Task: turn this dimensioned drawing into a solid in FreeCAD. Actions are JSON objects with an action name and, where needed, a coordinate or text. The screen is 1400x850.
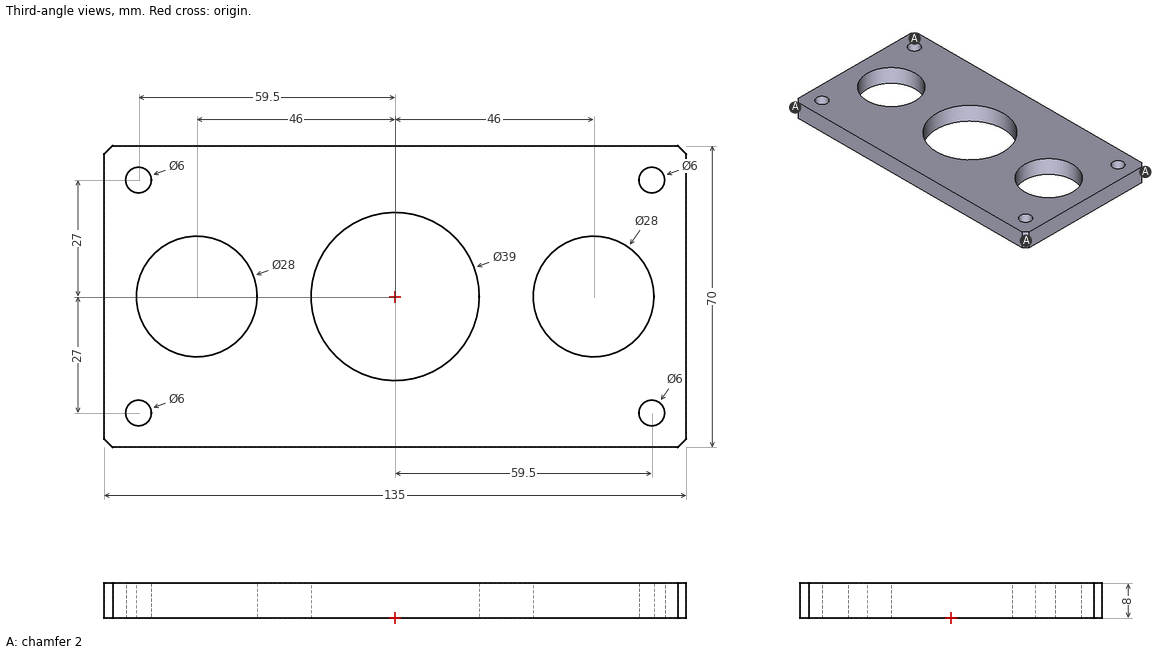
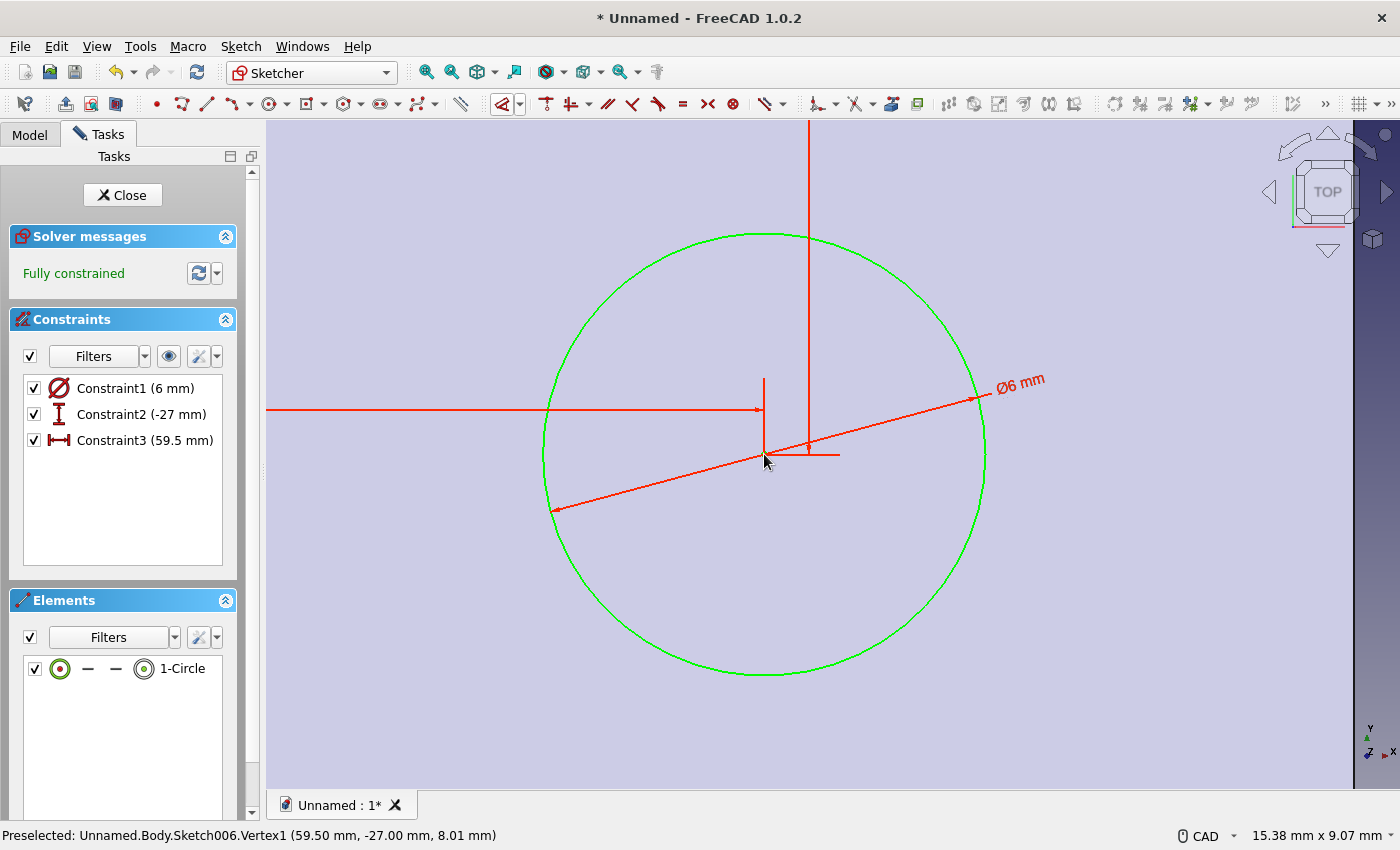
{"action": "left_click", "coordinate": [123, 195]}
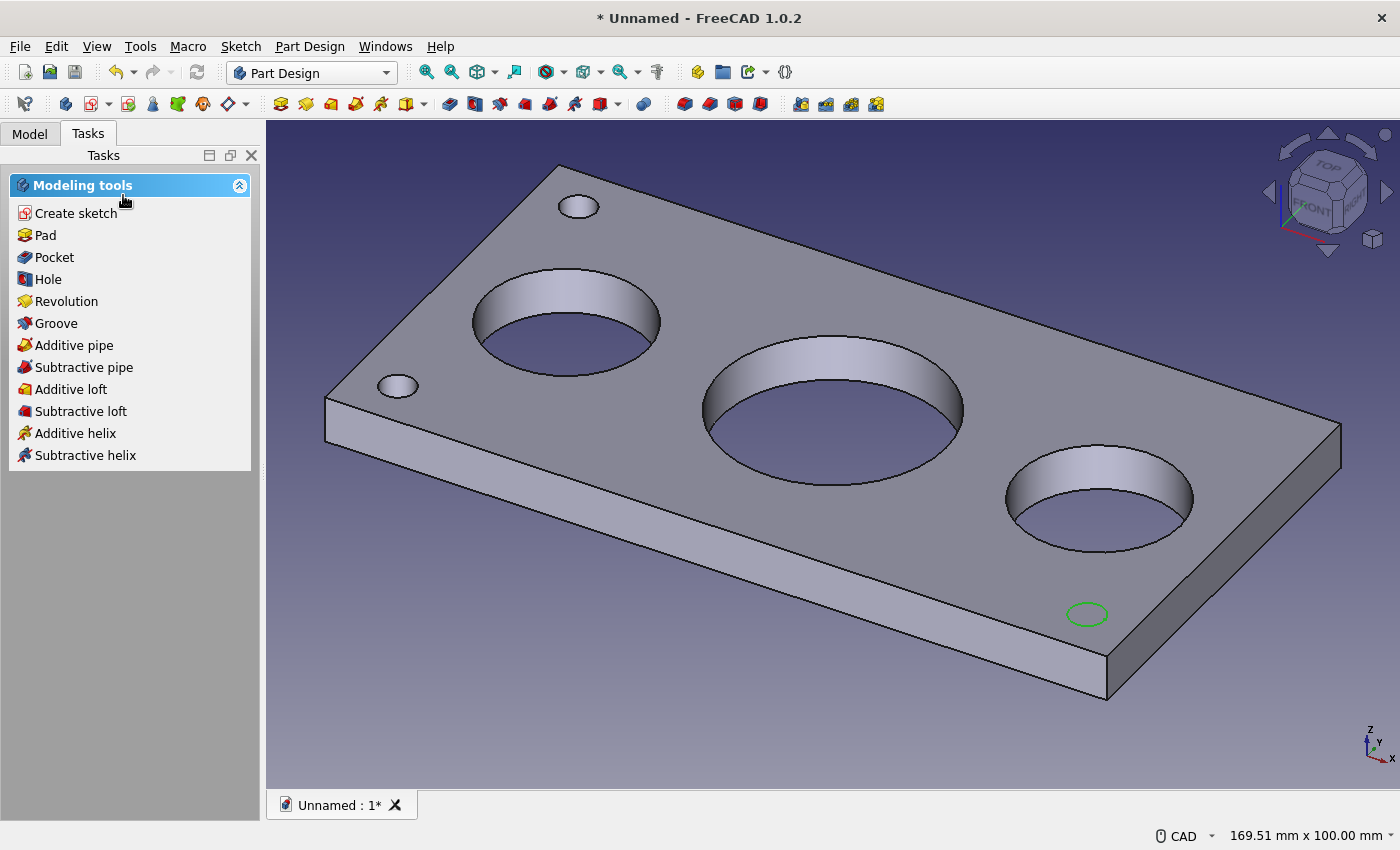
{"action": "left_click", "coordinate": [450, 104]}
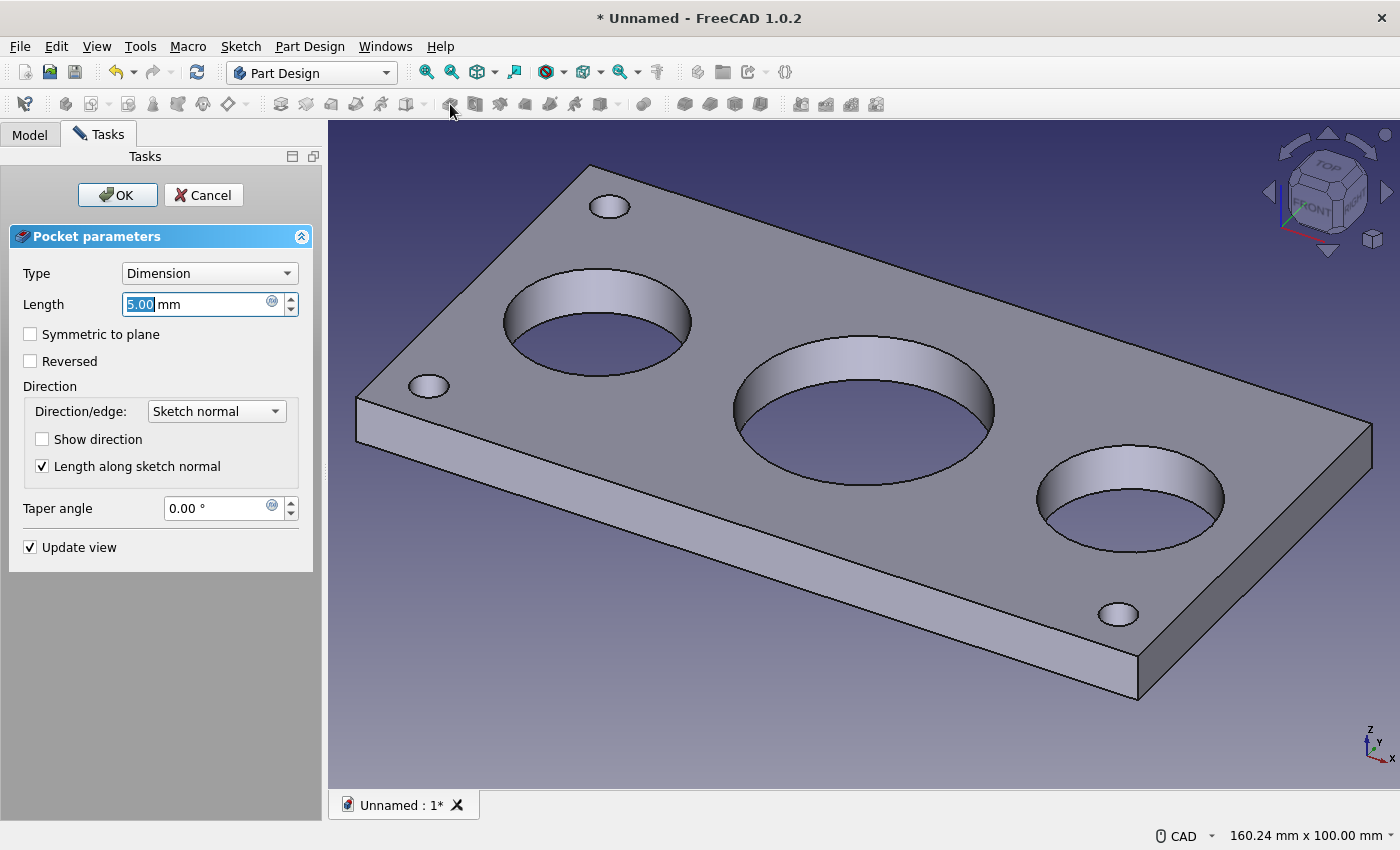
{"action": "left_click", "coordinate": [210, 274]}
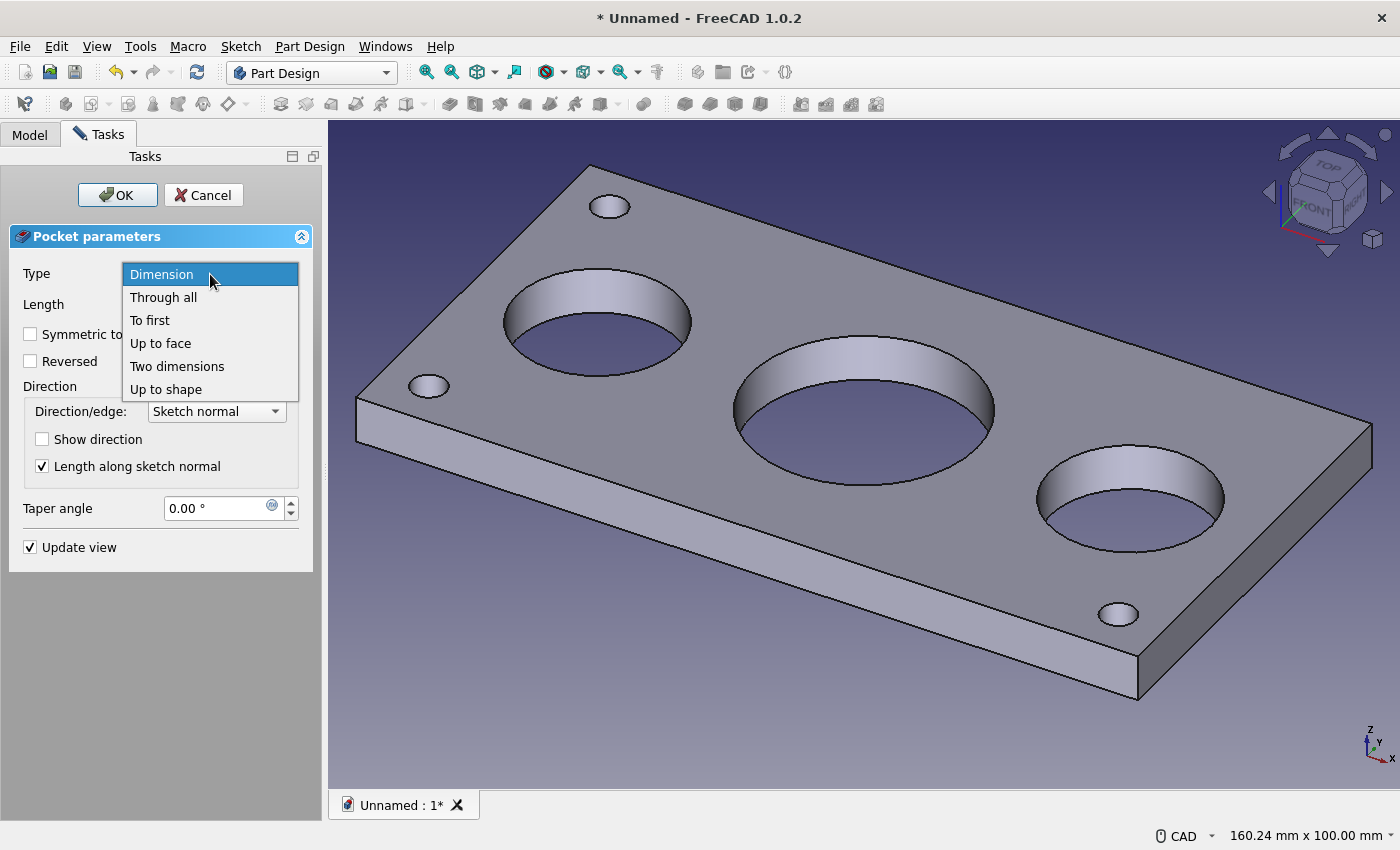
{"action": "left_click", "coordinate": [208, 320]}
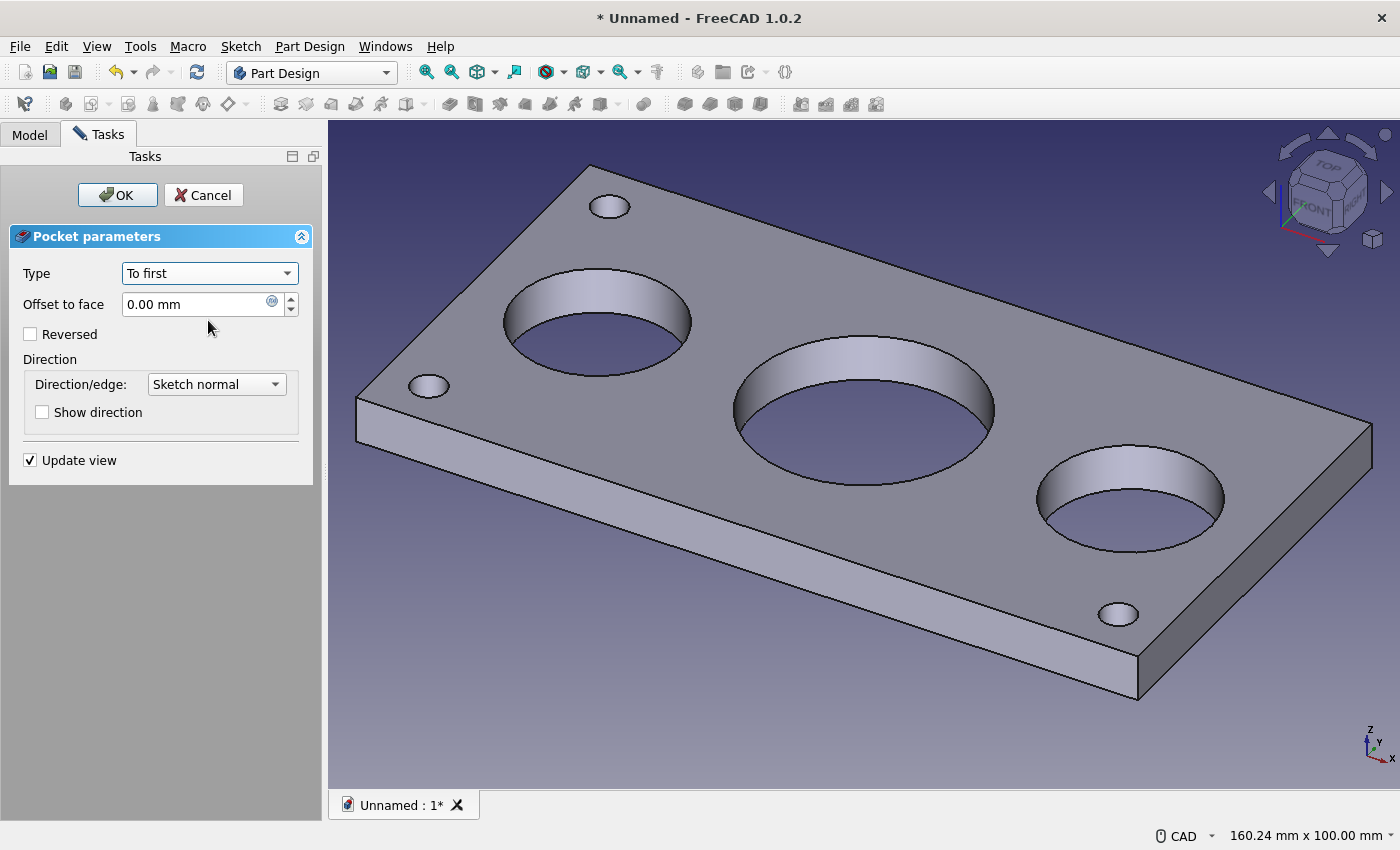
{"action": "left_click", "coordinate": [118, 195]}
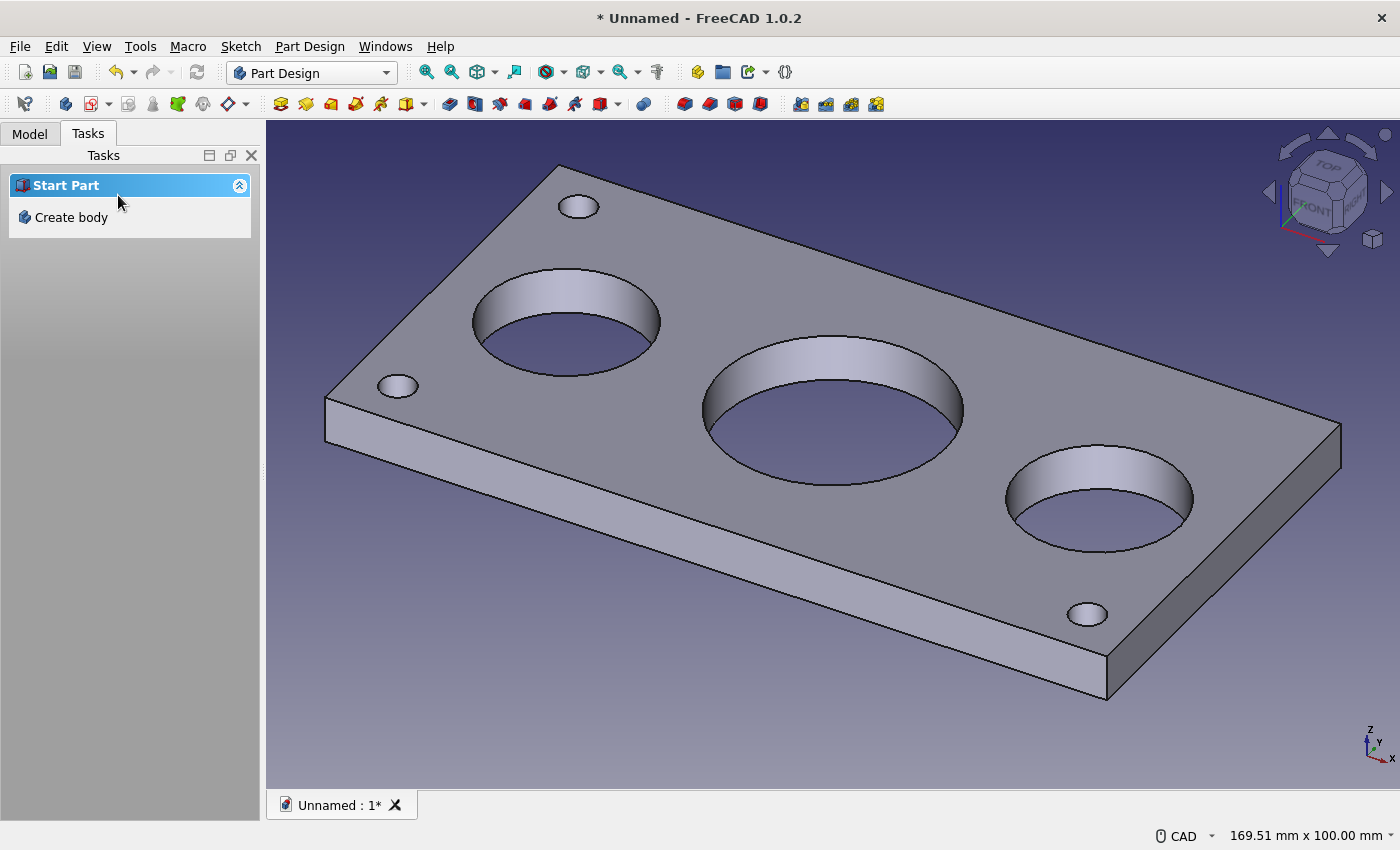
{"action": "left_click", "coordinate": [1235, 454]}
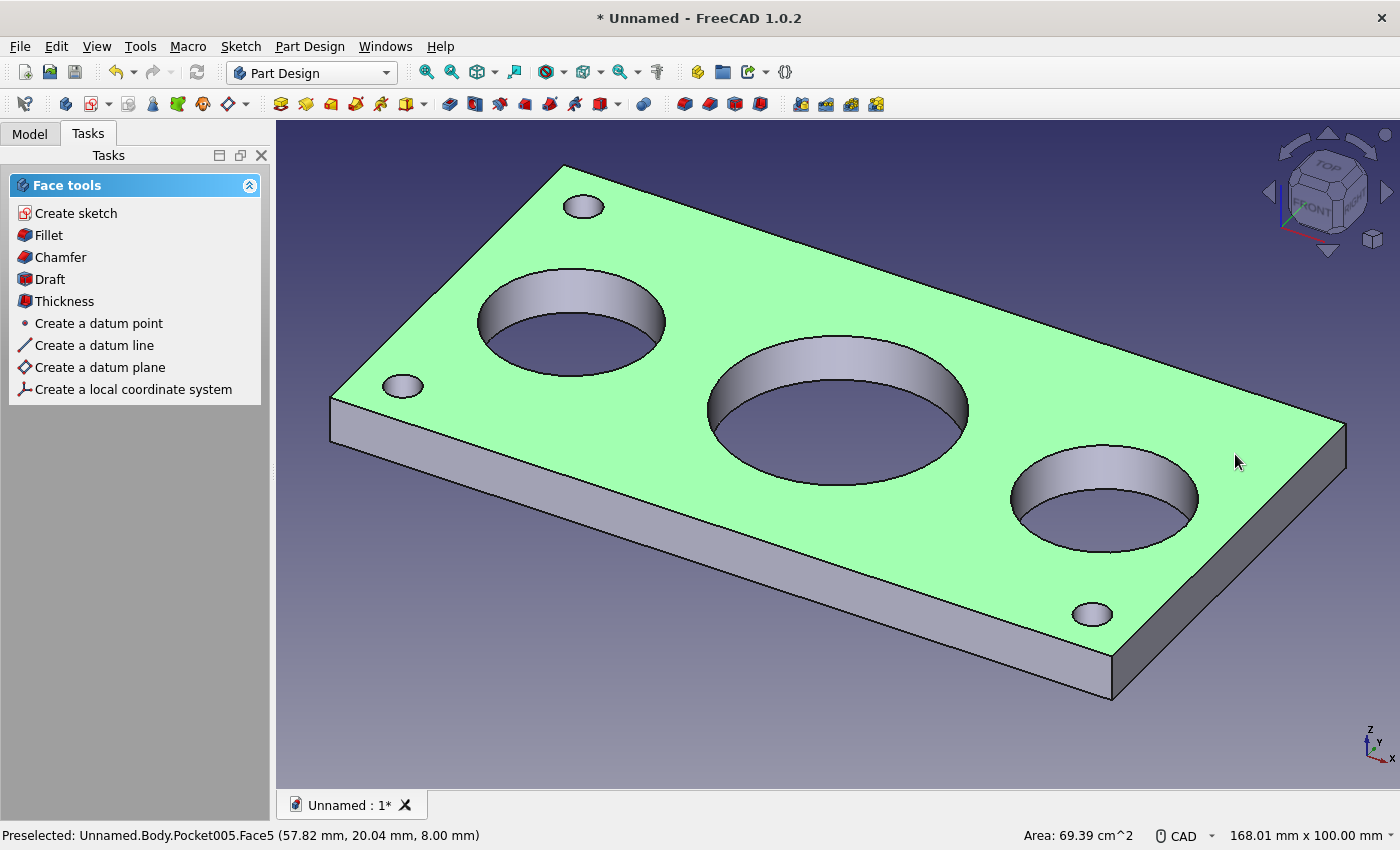
{"action": "left_click", "coordinate": [90, 104]}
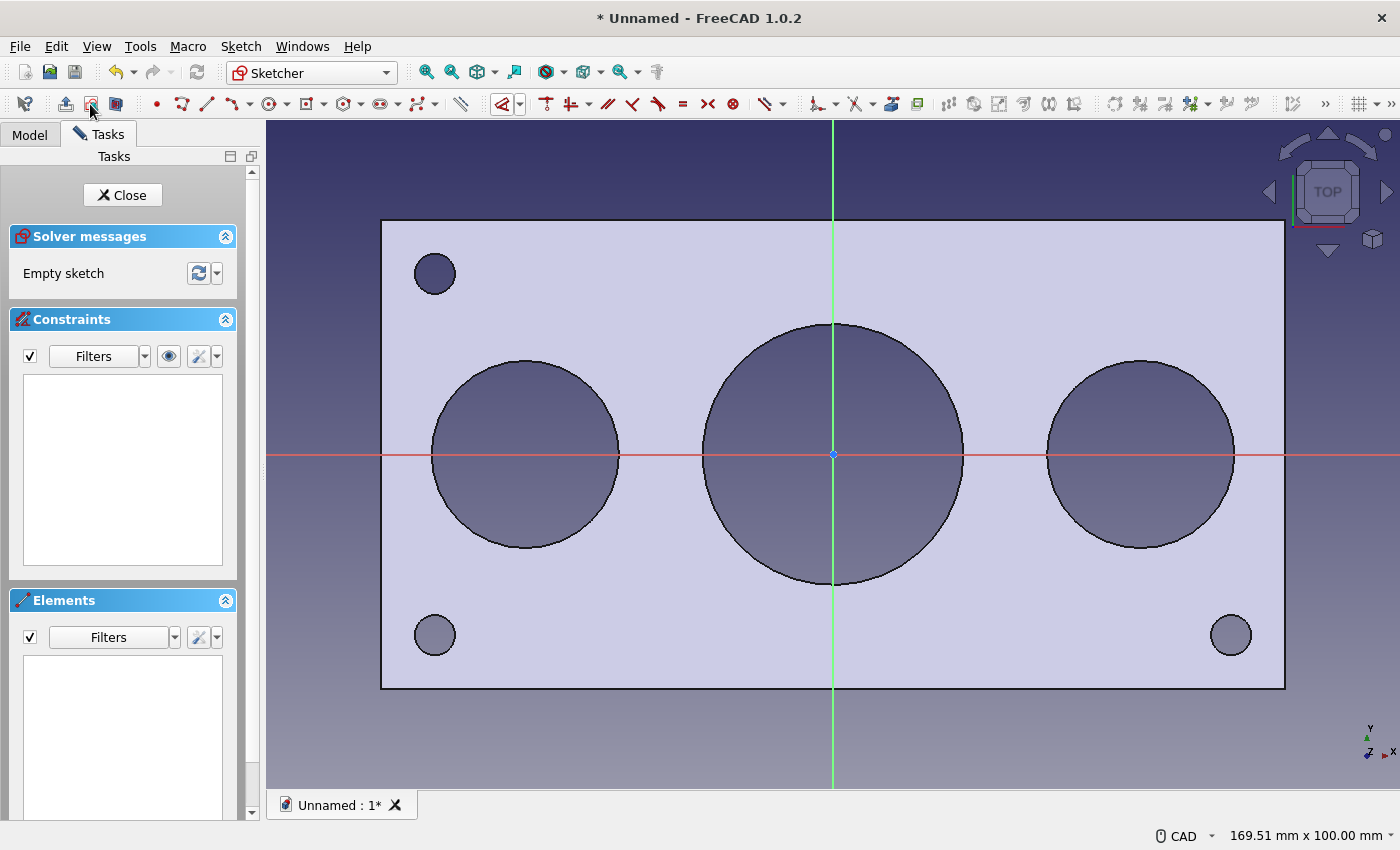
{"action": "scroll", "coordinate": [764, 454], "scroll_direction": "down", "scroll_amount": 5}